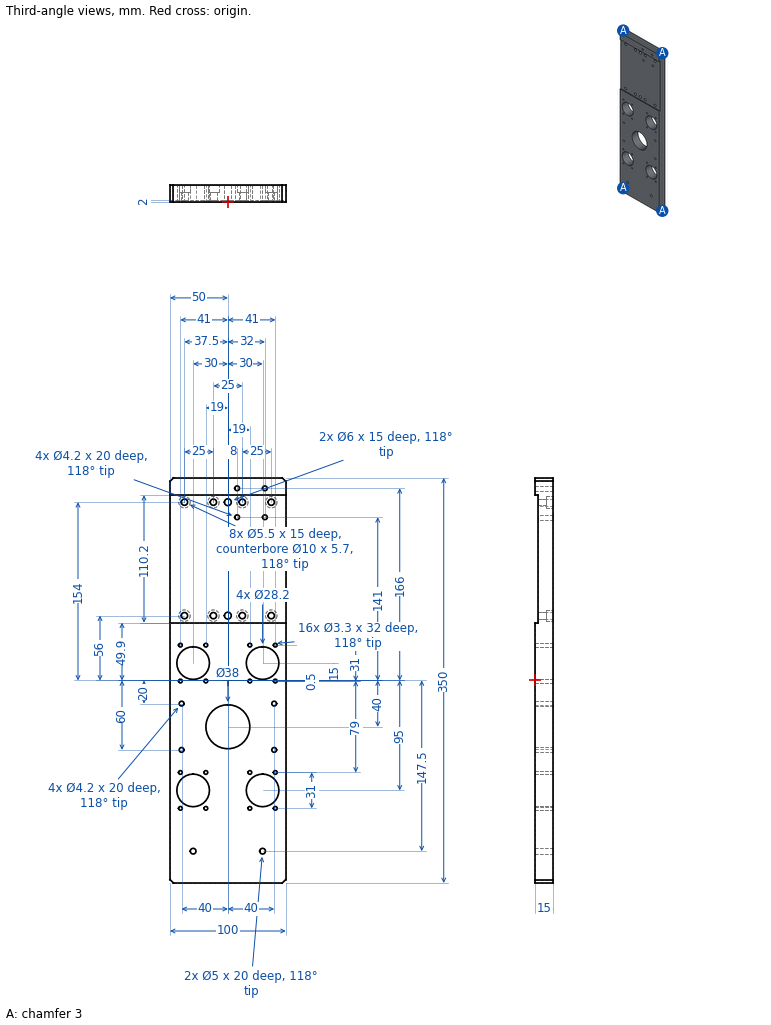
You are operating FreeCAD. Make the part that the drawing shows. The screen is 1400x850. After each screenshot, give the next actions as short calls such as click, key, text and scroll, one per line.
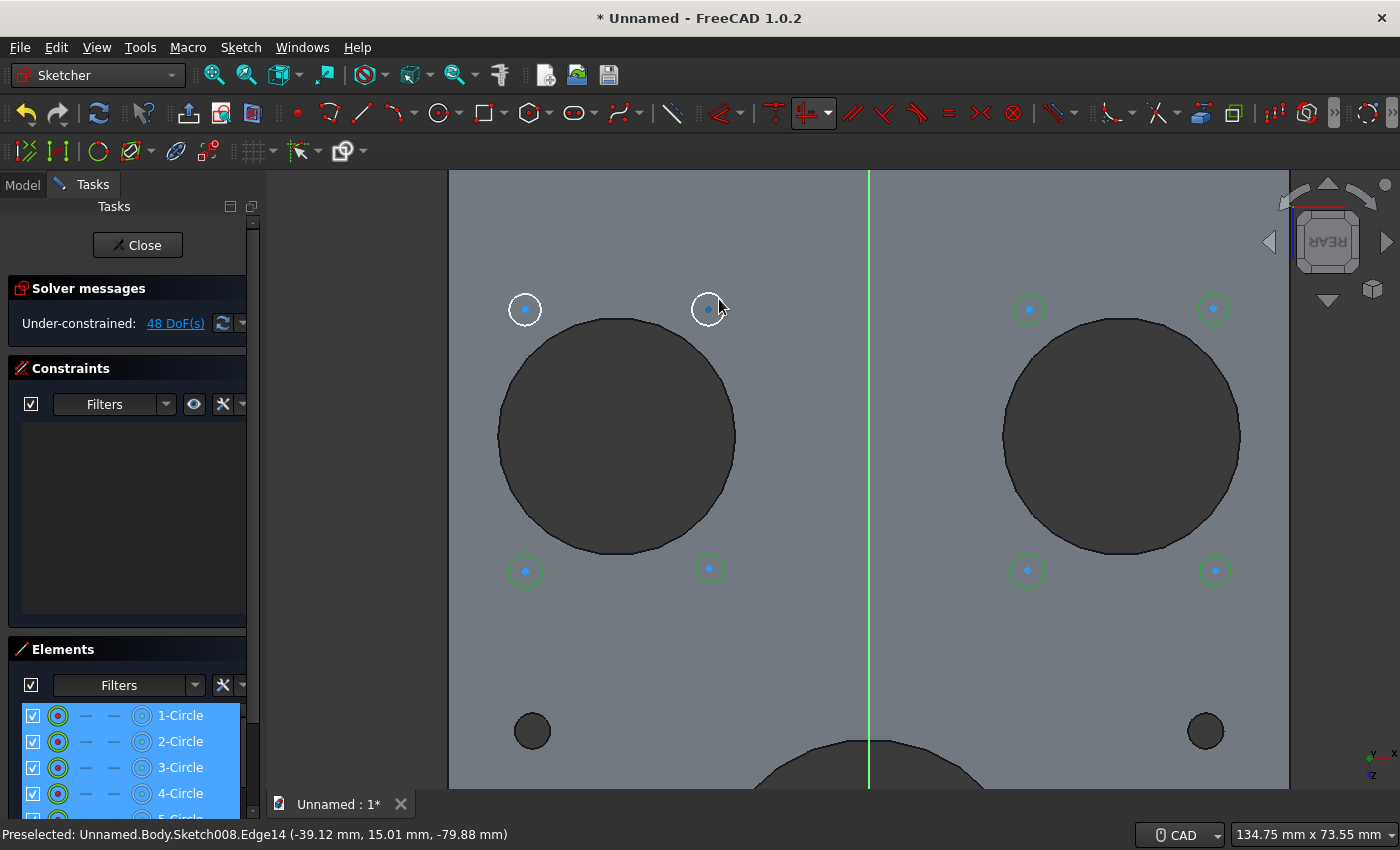
click(720, 298)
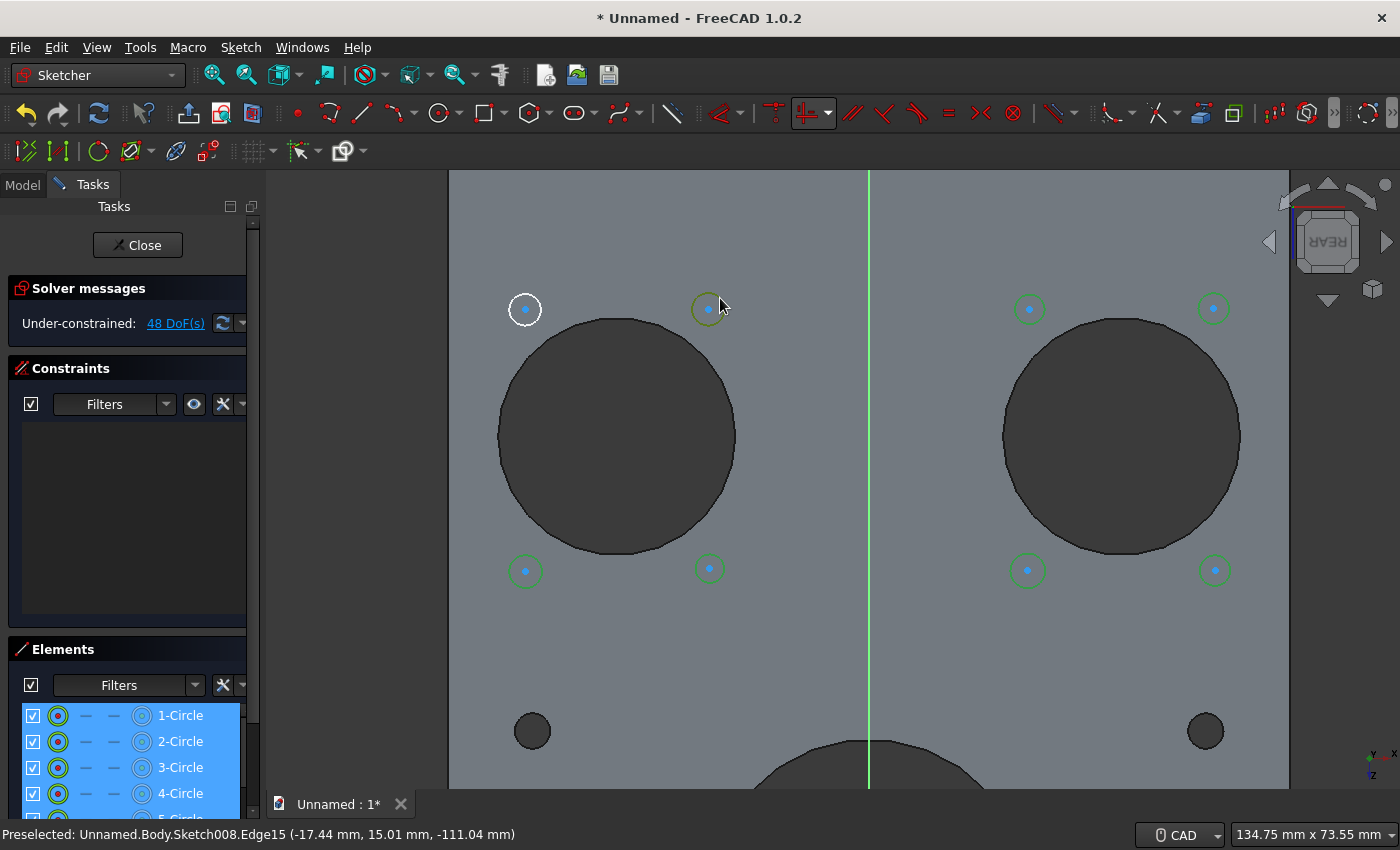
click(536, 299)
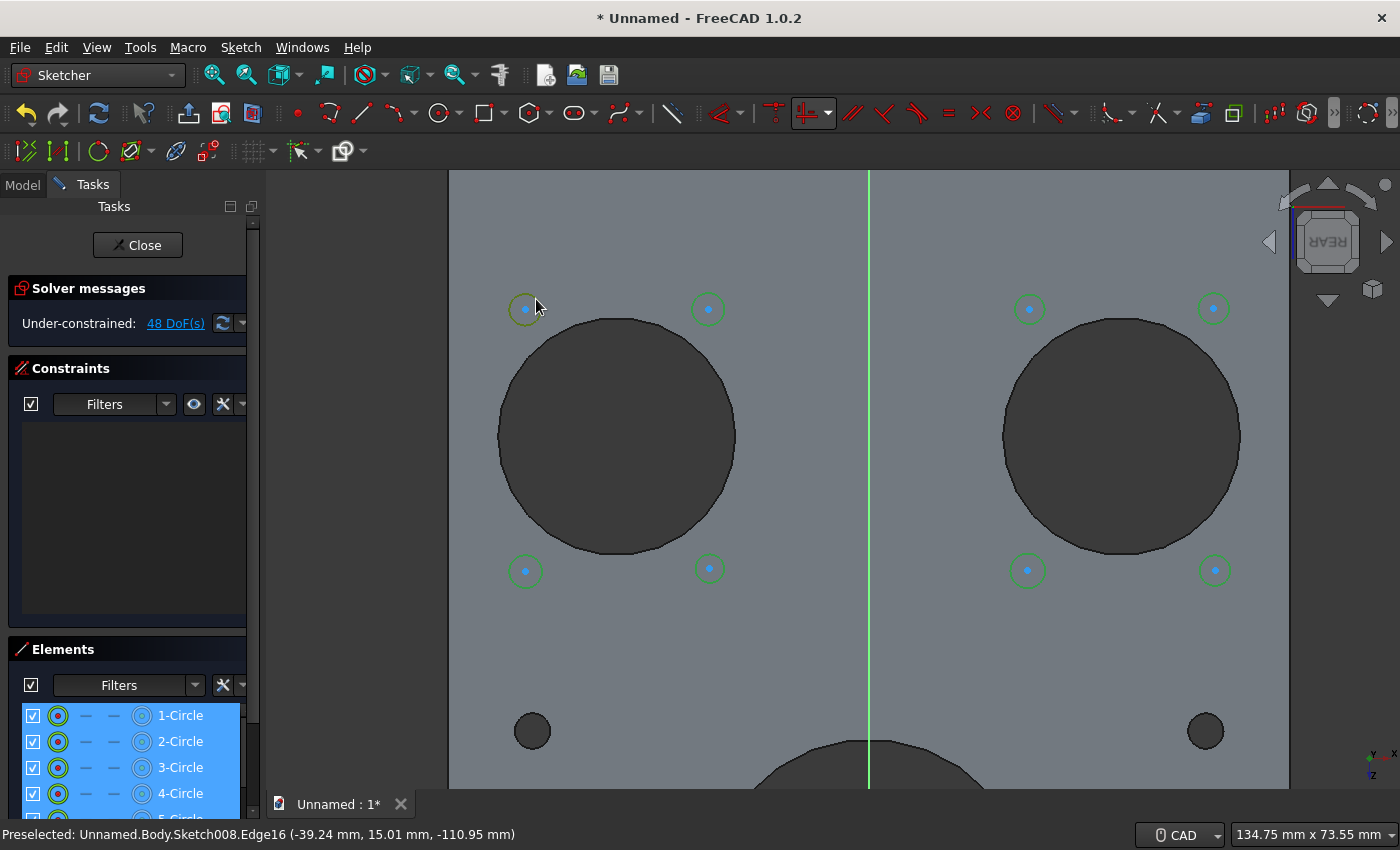
key(e)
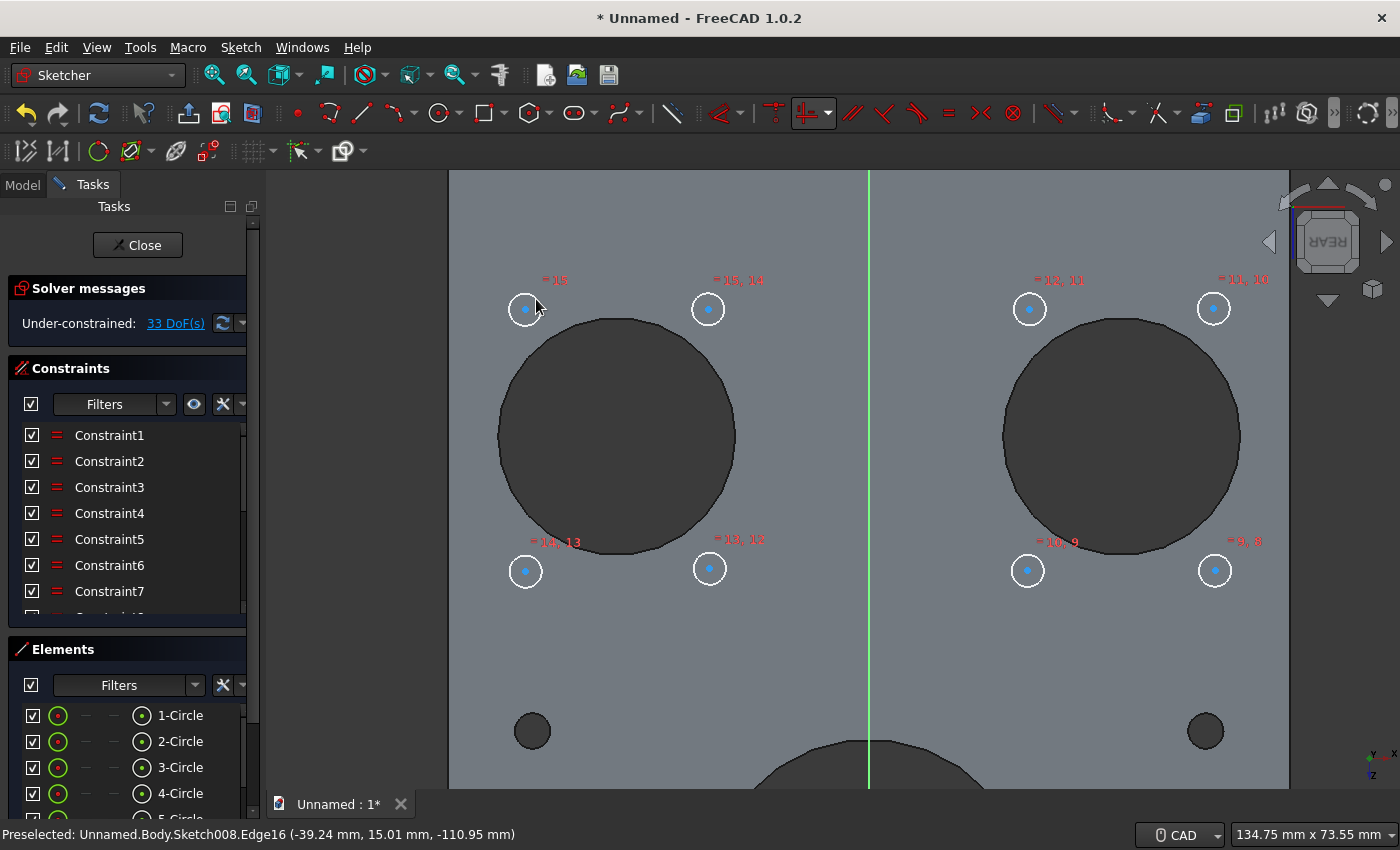
scroll(719, 299, down, 6)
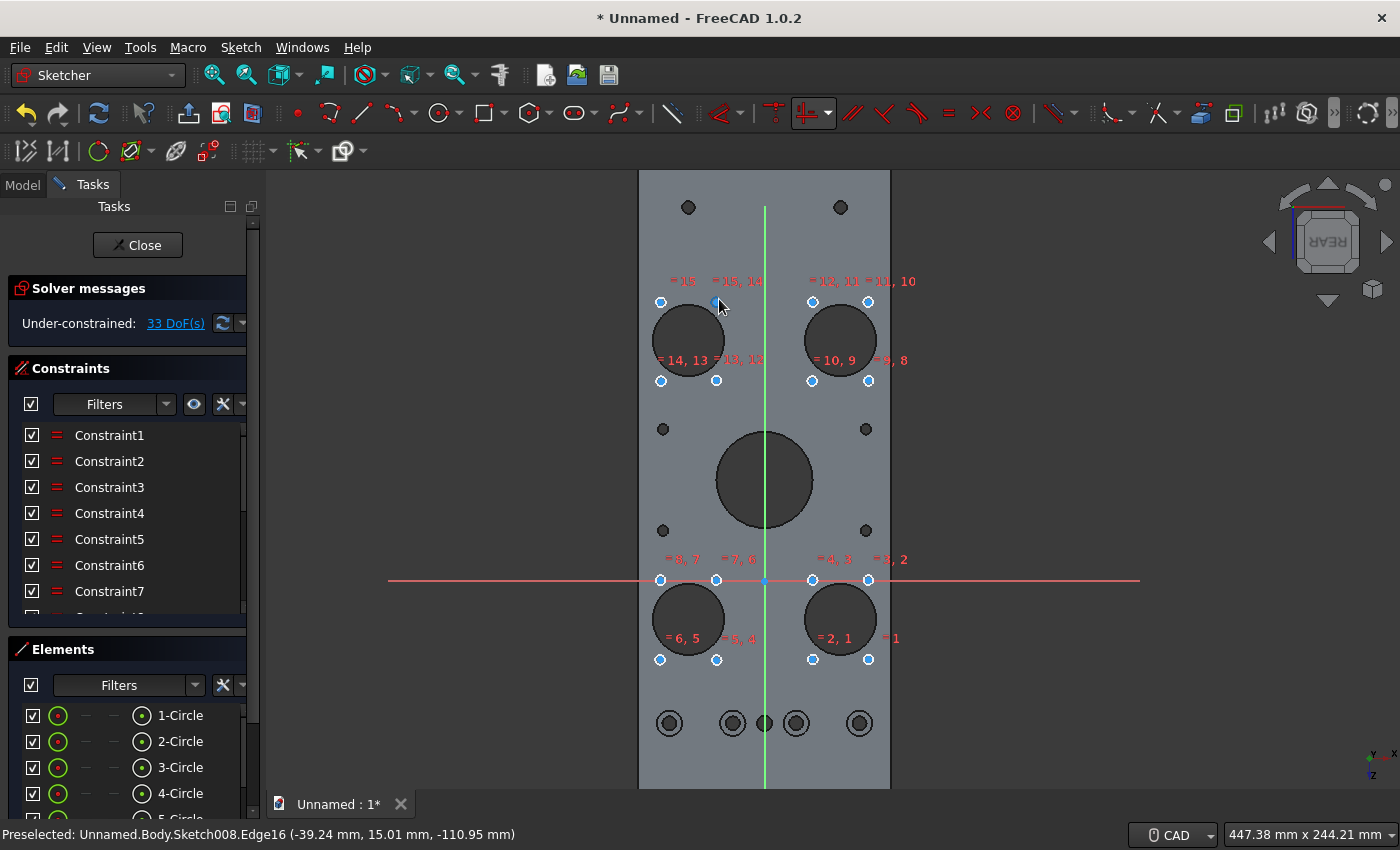
click(868, 660)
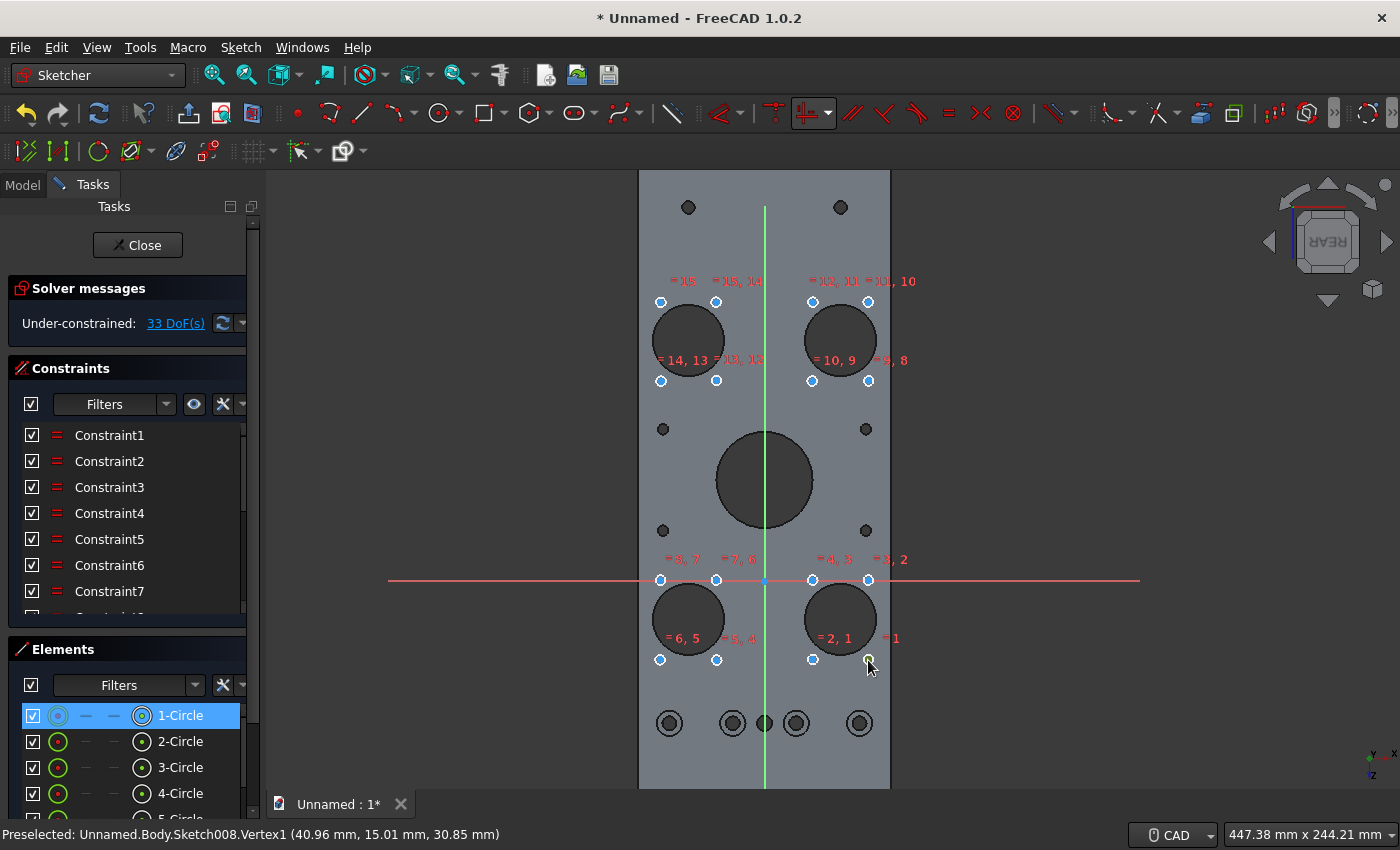
click(813, 660)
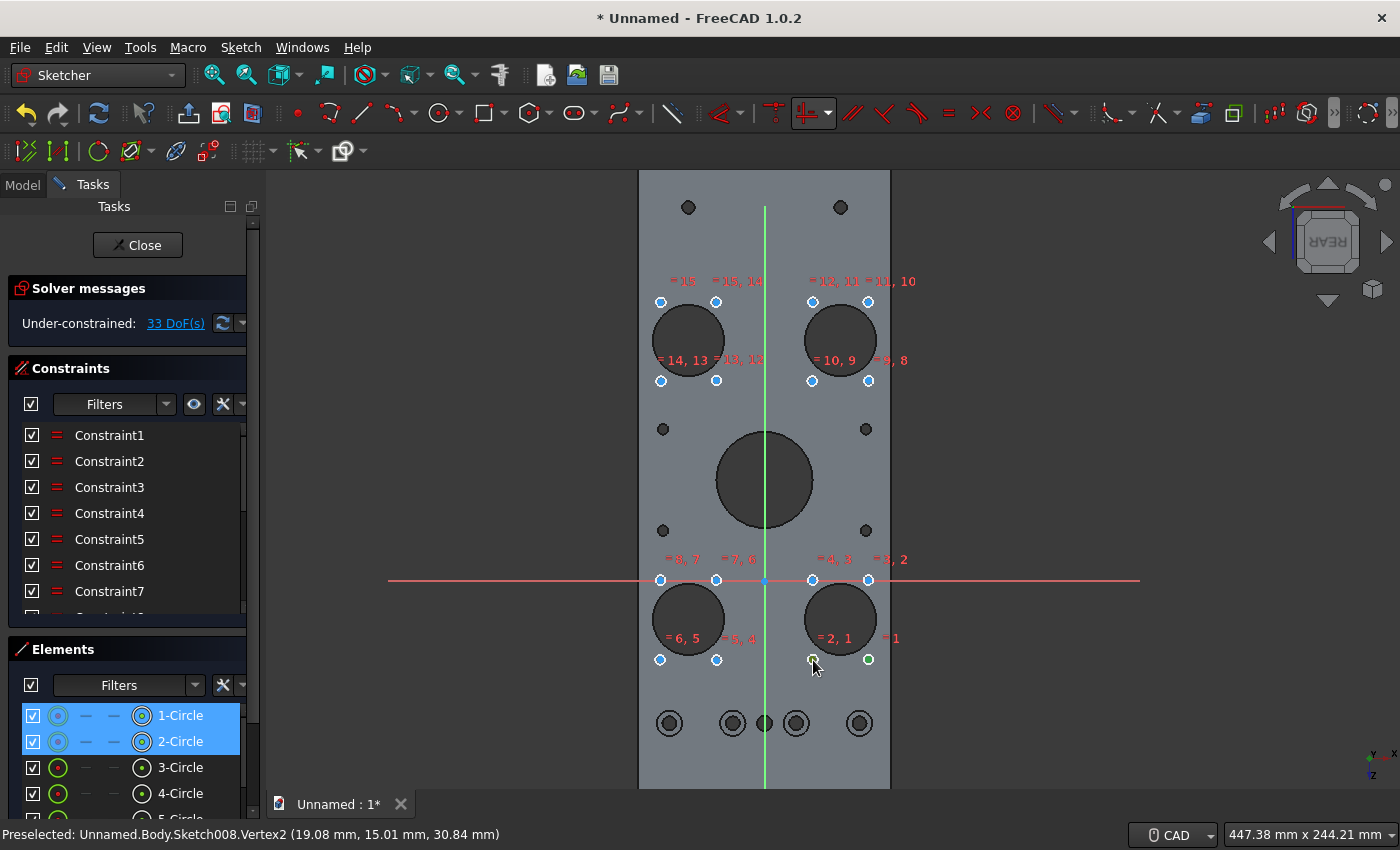
click(830, 114)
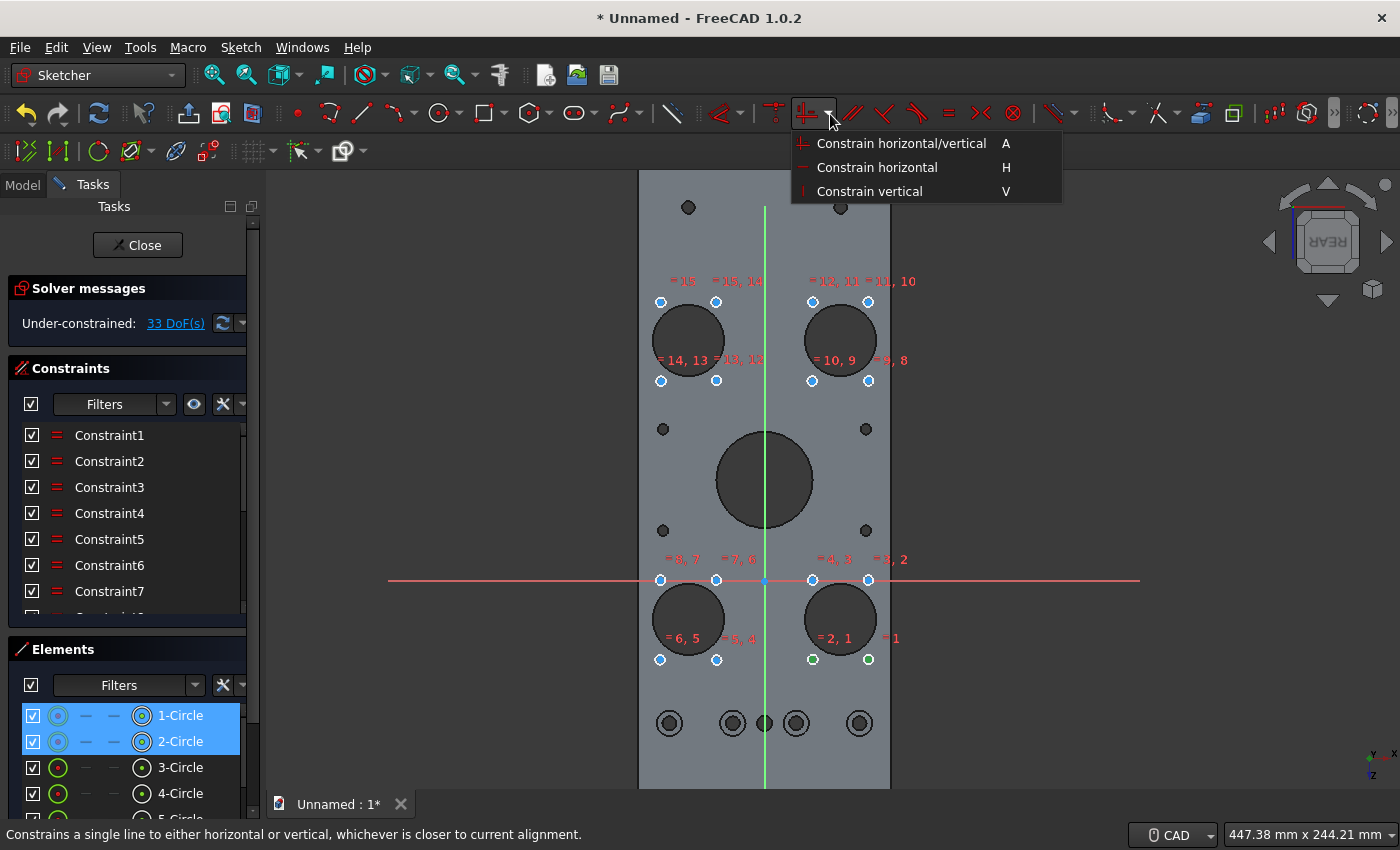
click(927, 167)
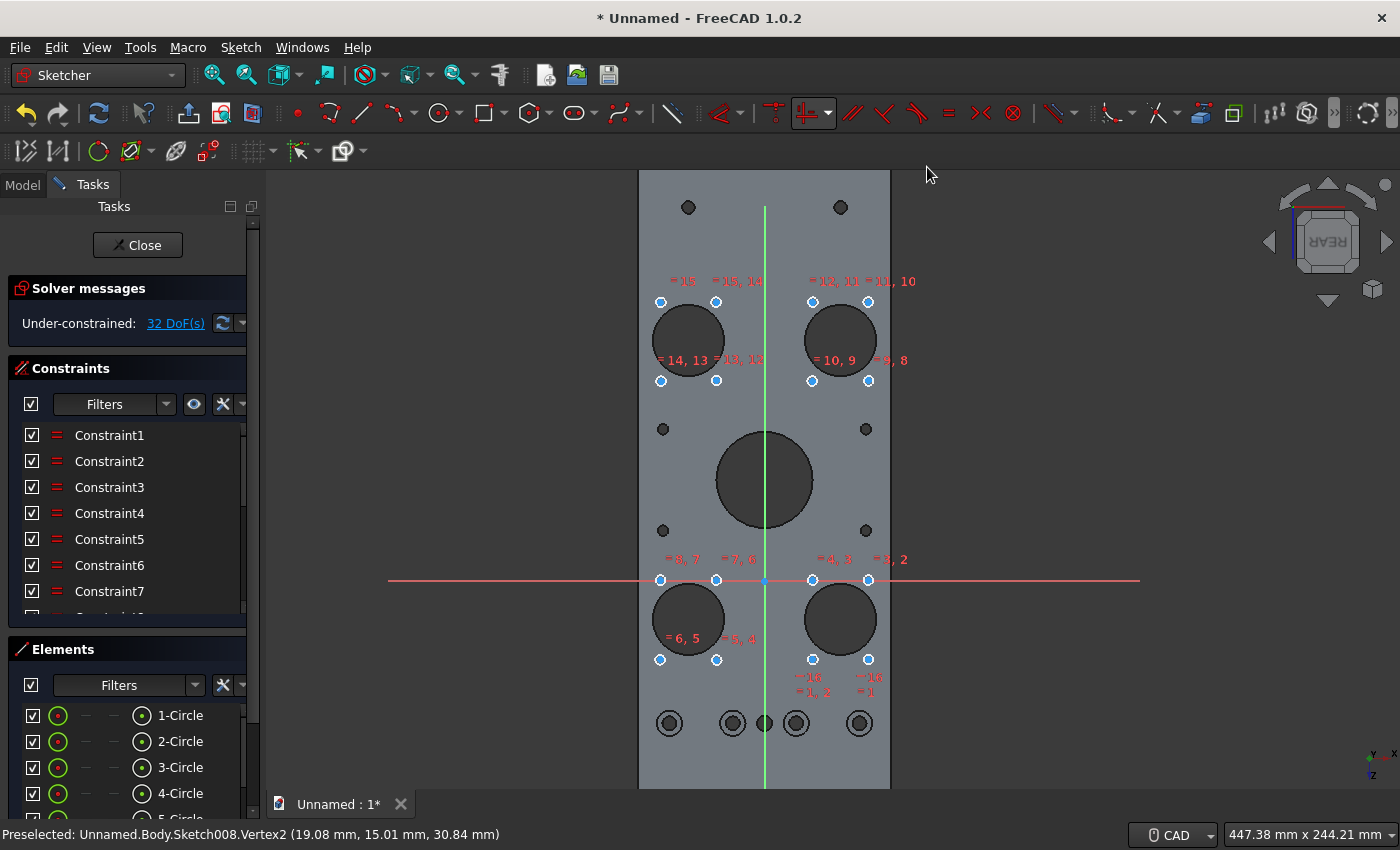
click(868, 660)